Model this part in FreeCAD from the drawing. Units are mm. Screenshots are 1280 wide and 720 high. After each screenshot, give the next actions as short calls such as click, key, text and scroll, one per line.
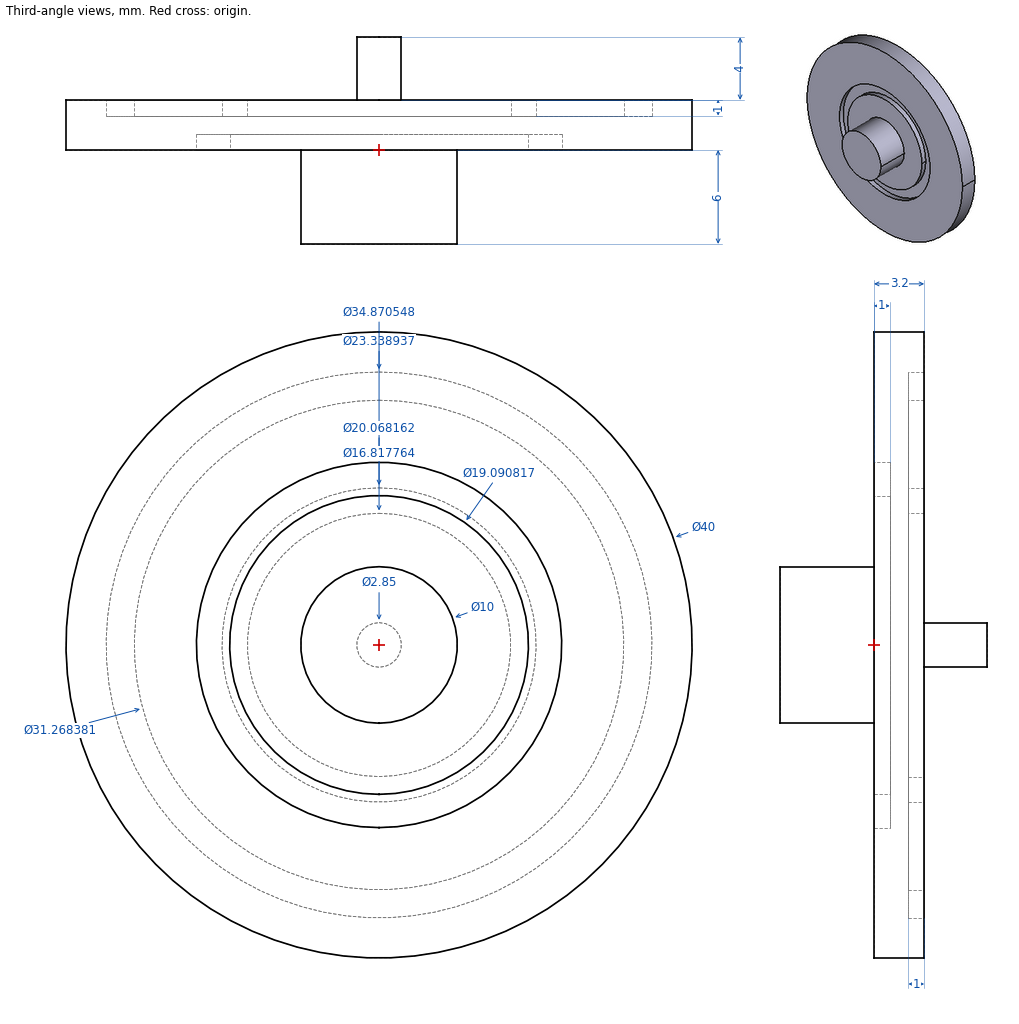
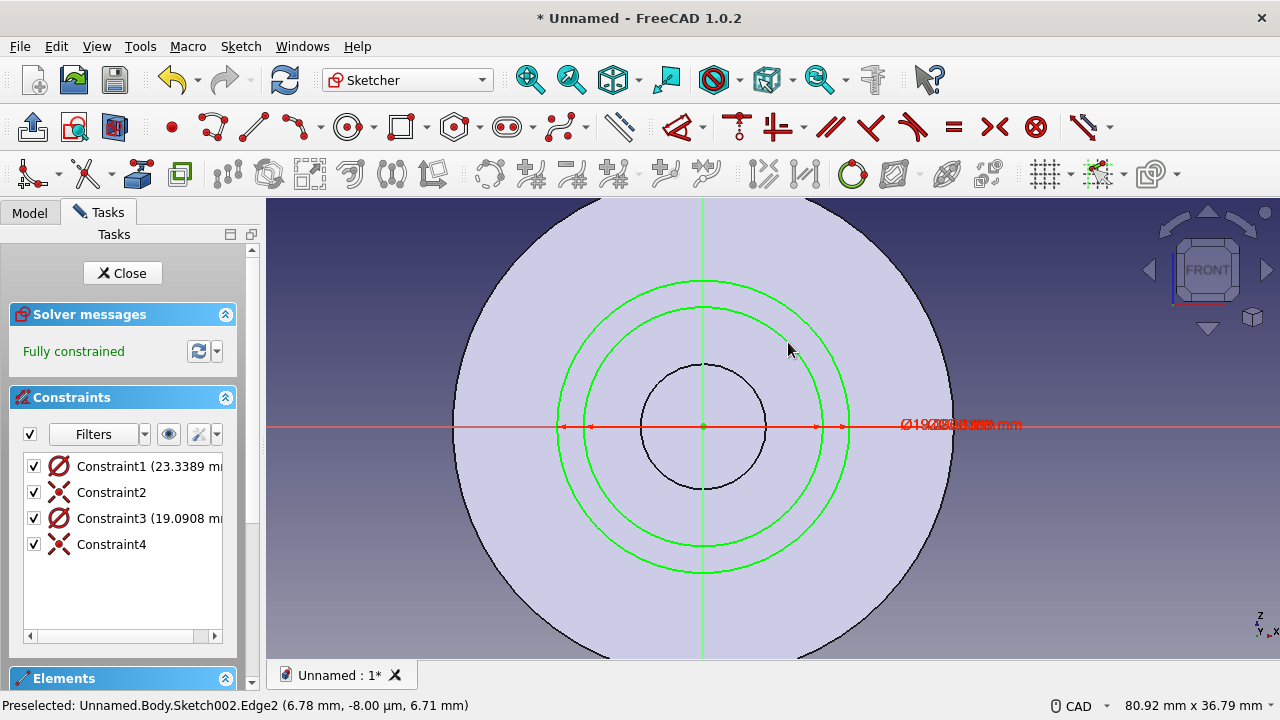
click(123, 273)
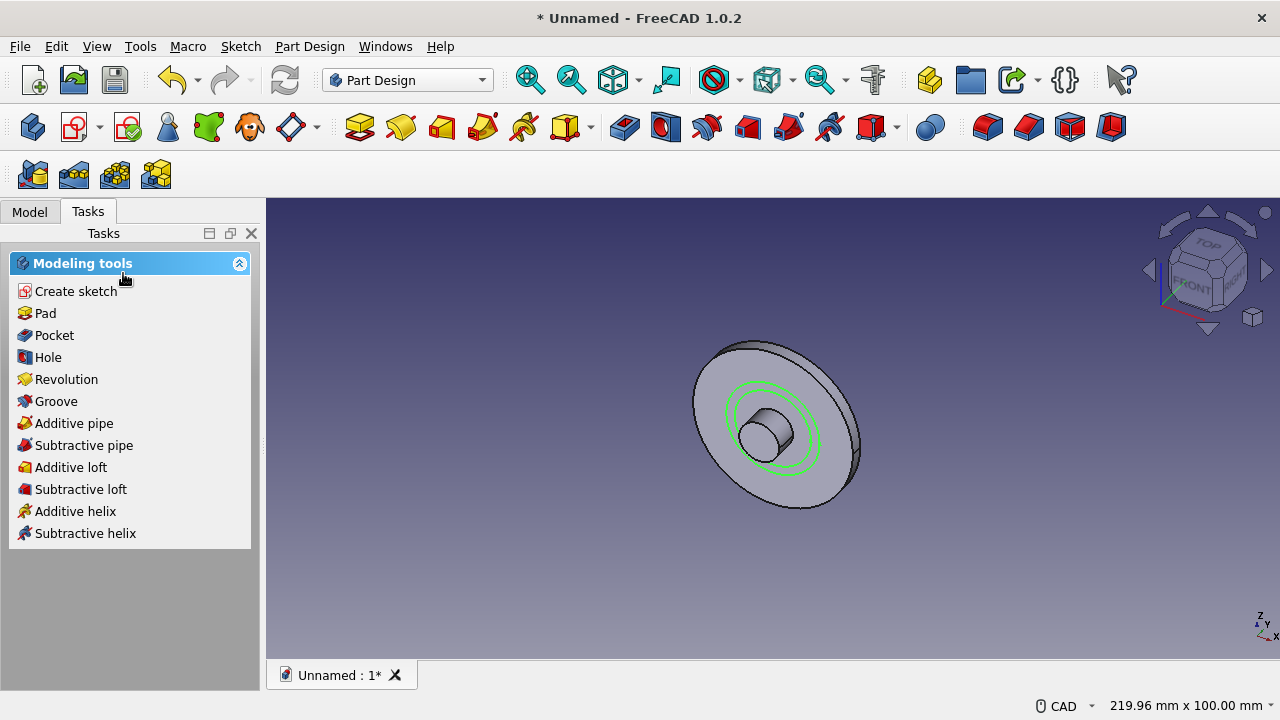
click(625, 128)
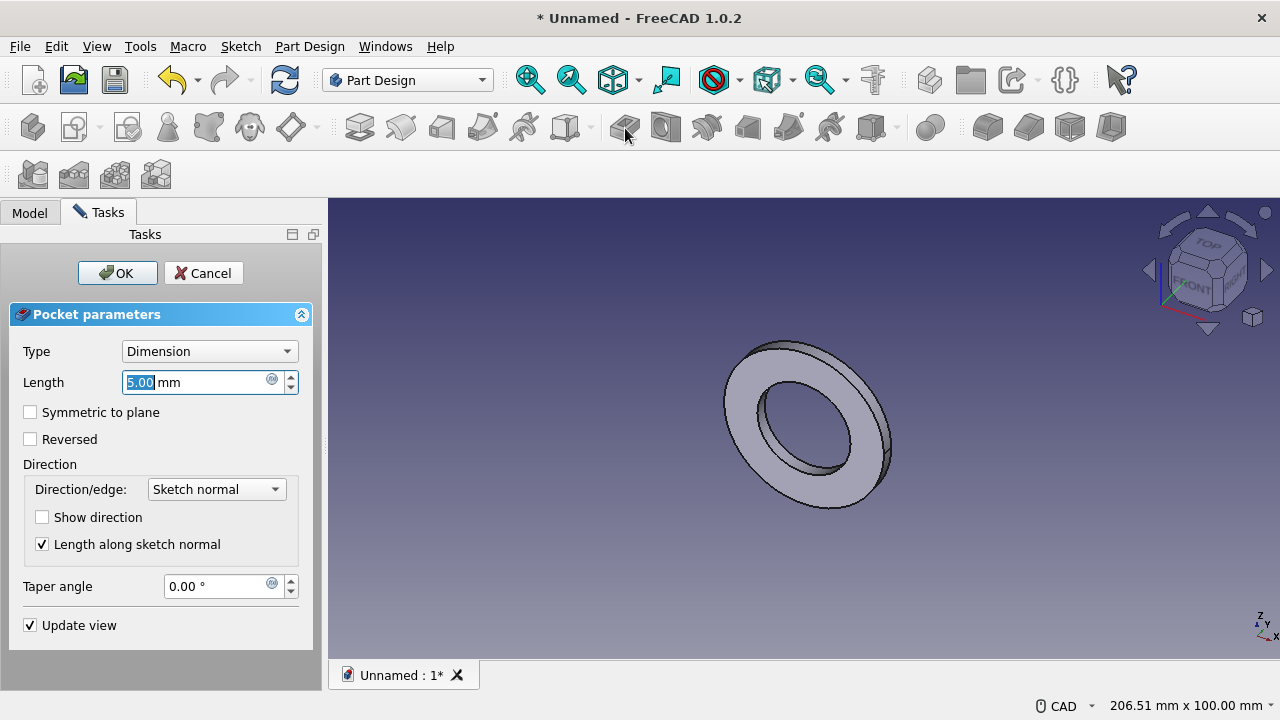
text(1)
key(Tab)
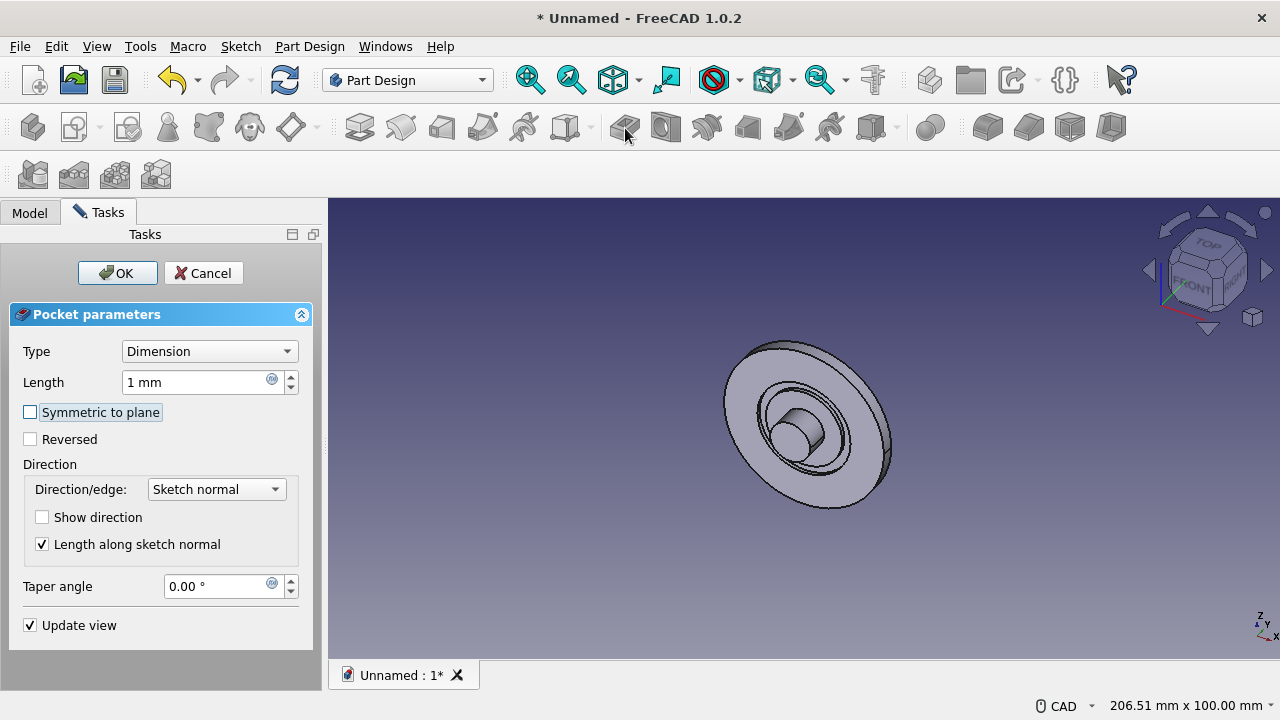
click(118, 273)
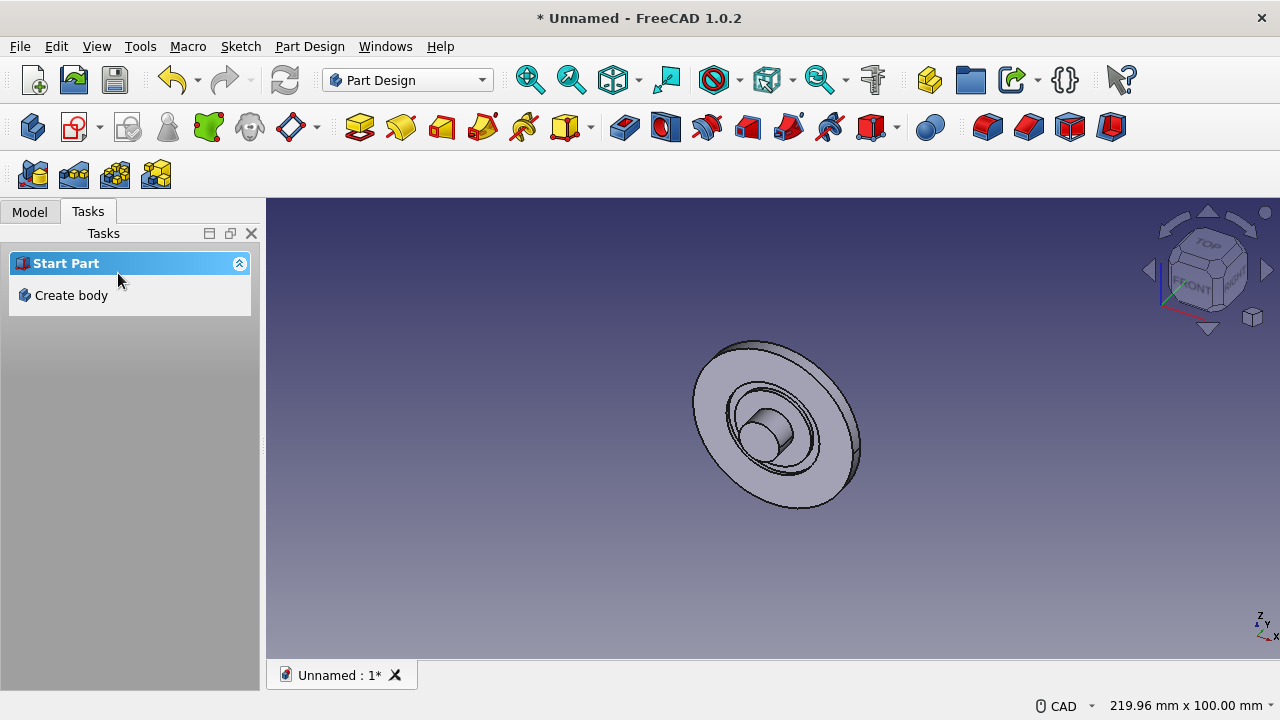
key(4)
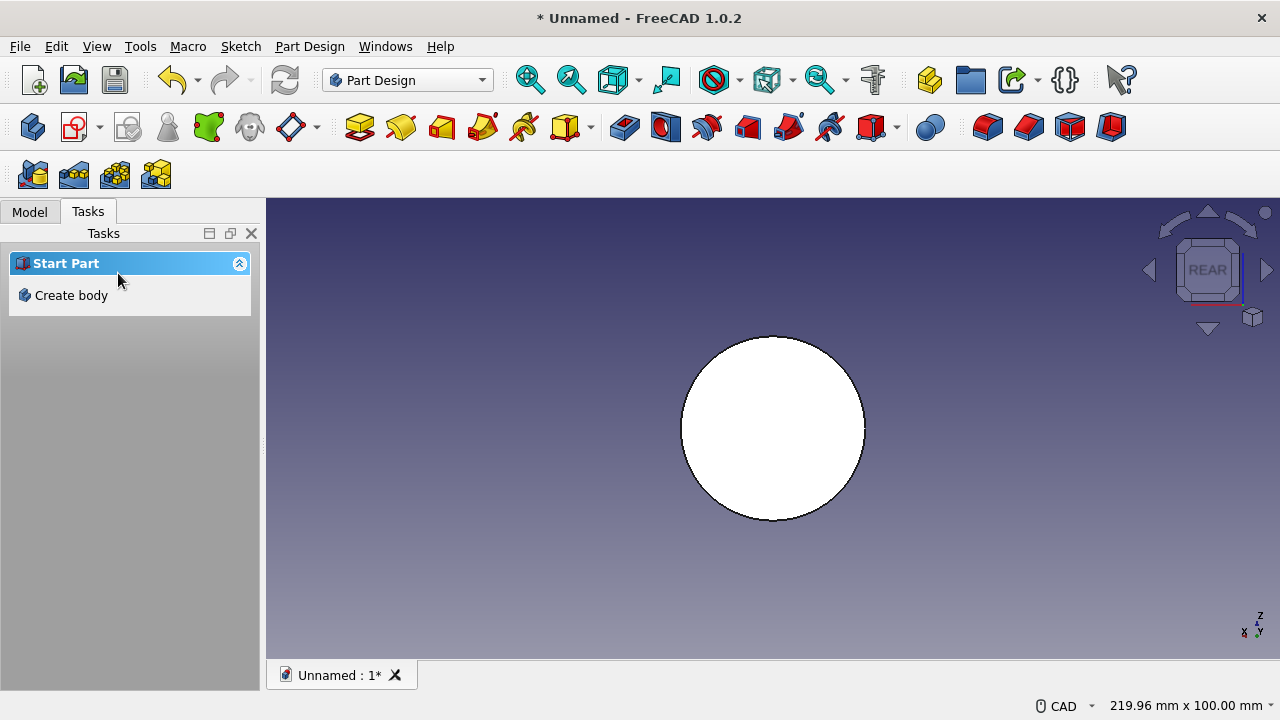
click(531, 80)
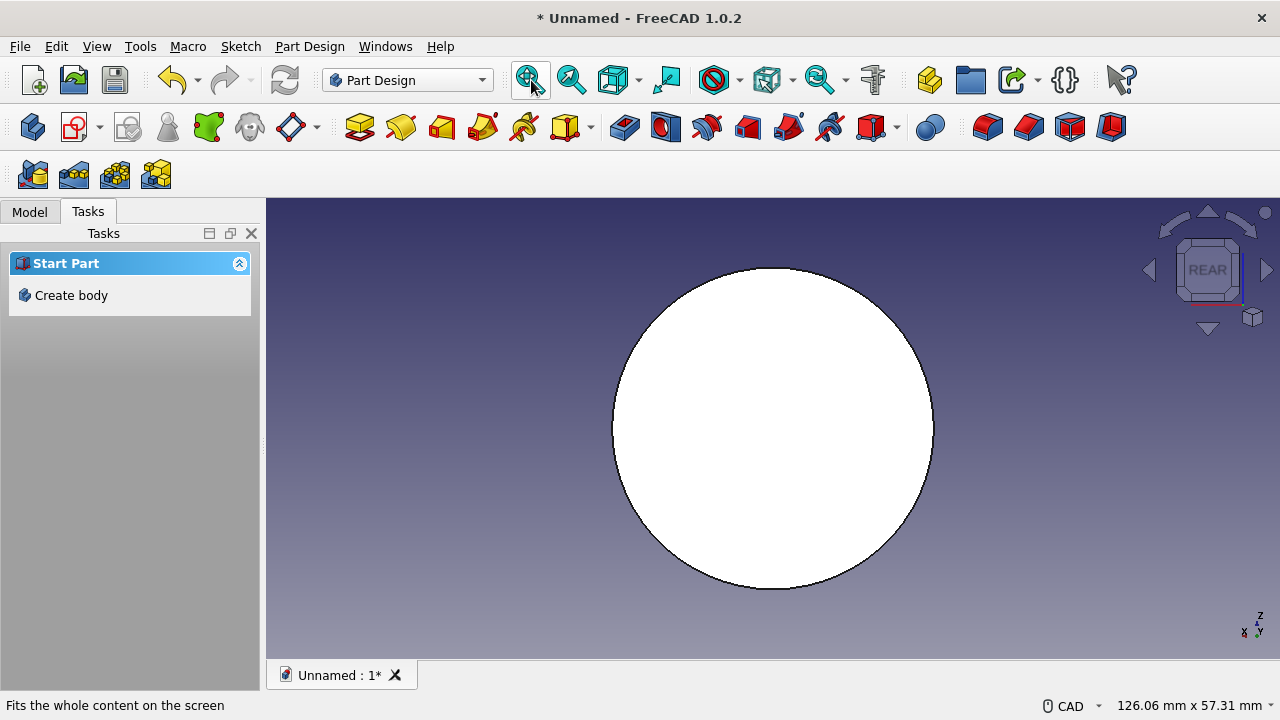
click(773, 428)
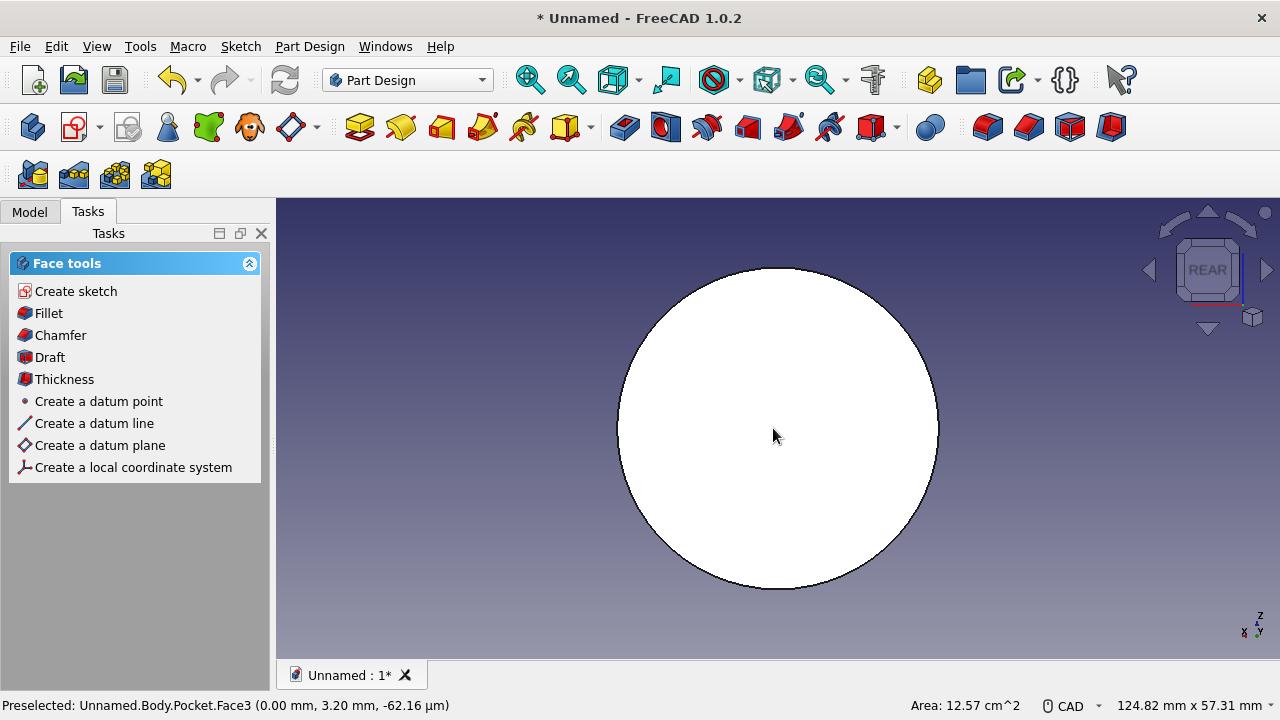
click(74, 128)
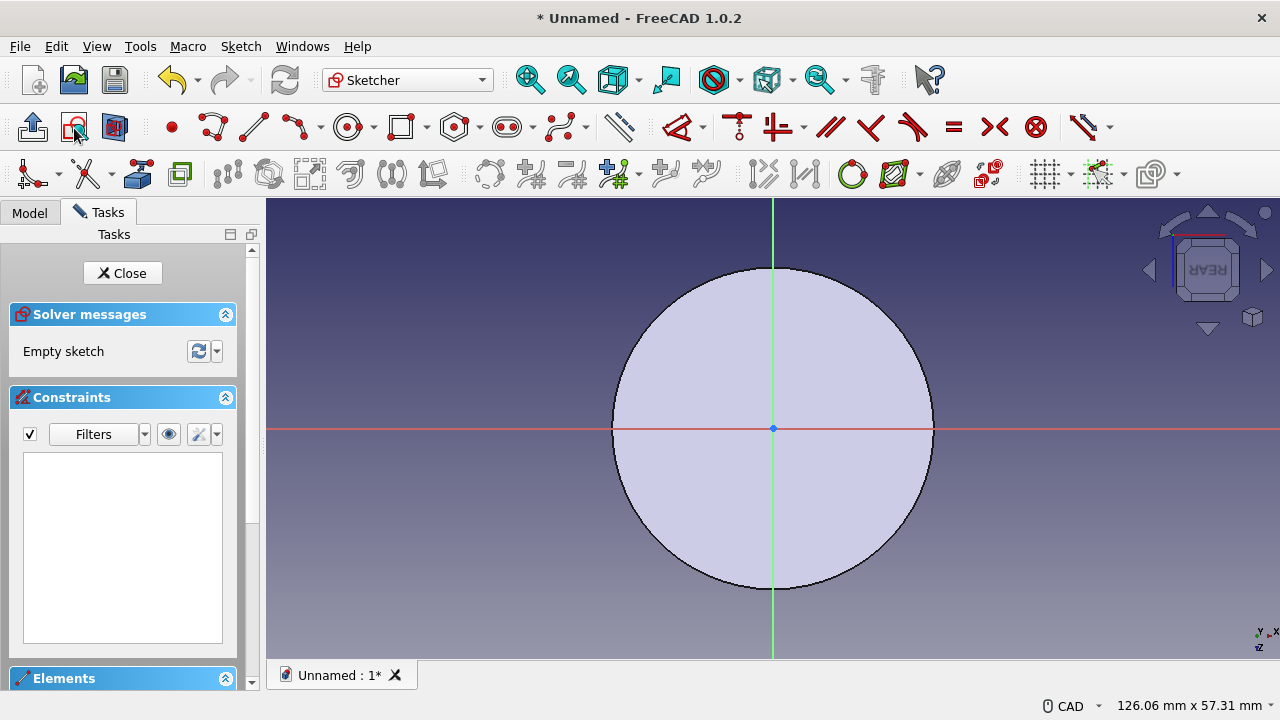
scroll(778, 428, up, 13)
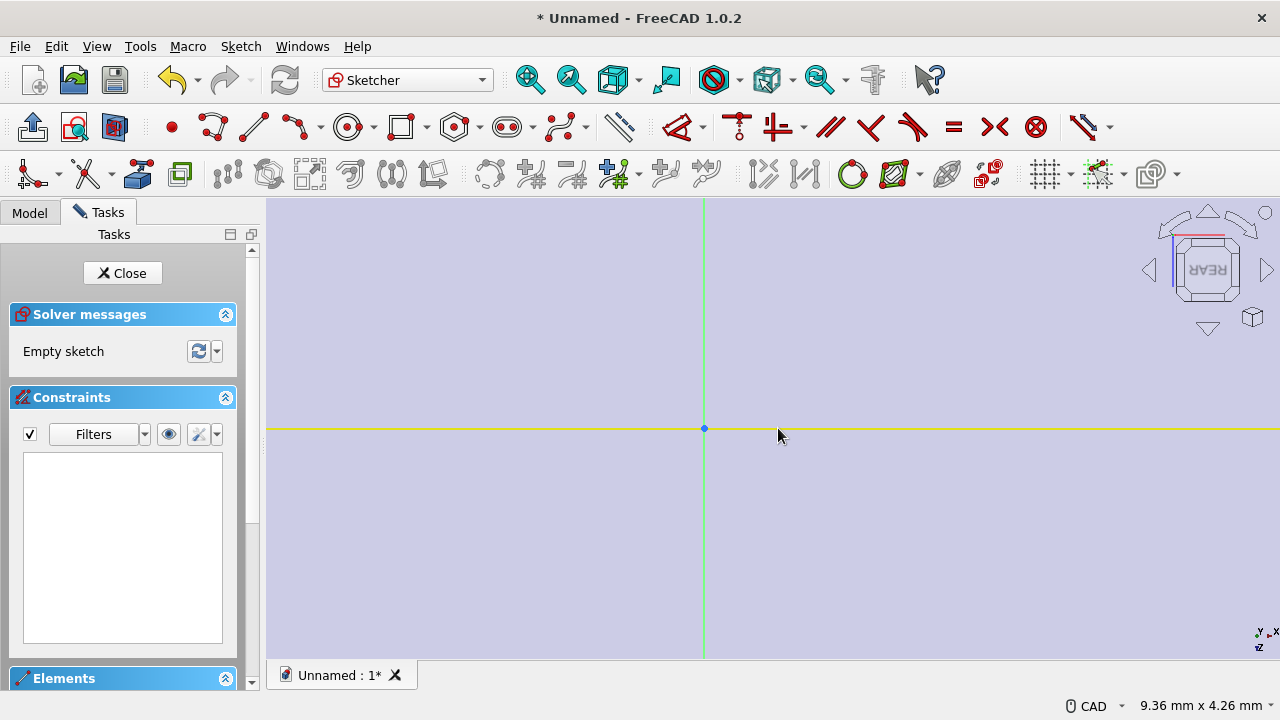
click(348, 128)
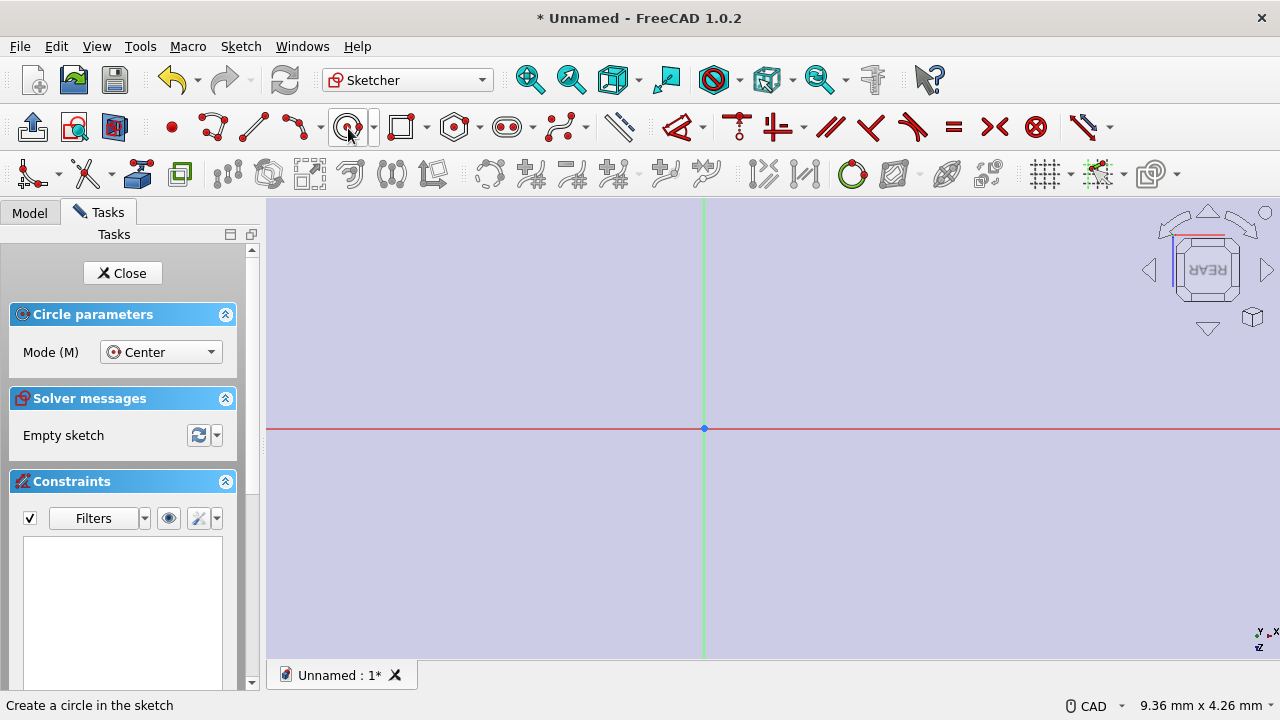
click(704, 428)
move(814, 319)